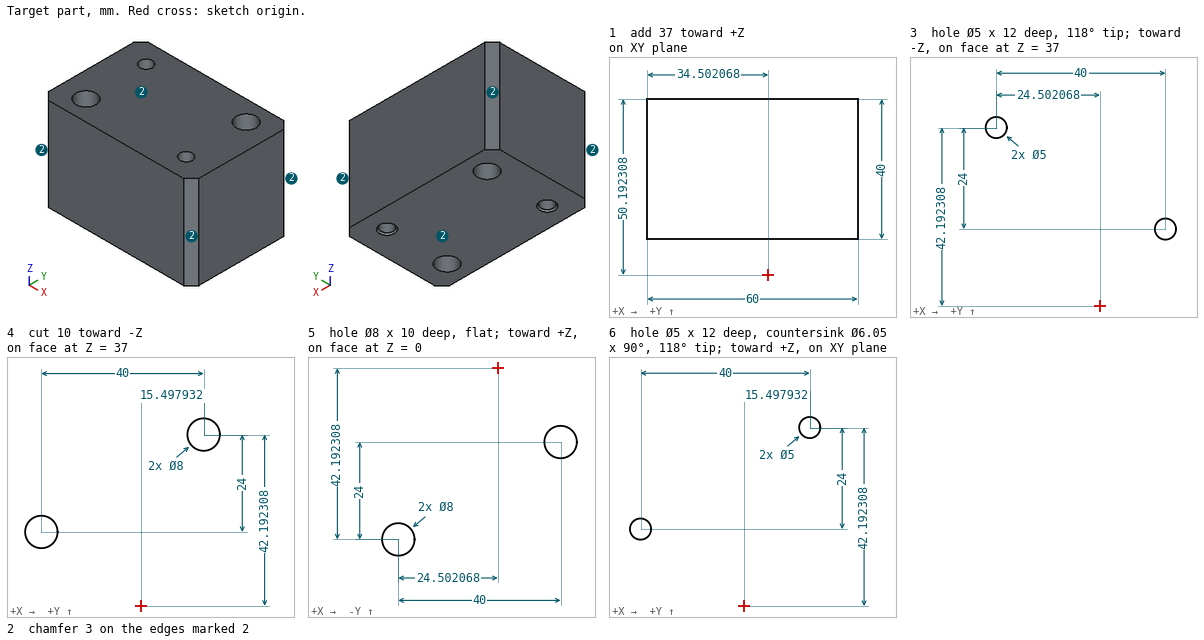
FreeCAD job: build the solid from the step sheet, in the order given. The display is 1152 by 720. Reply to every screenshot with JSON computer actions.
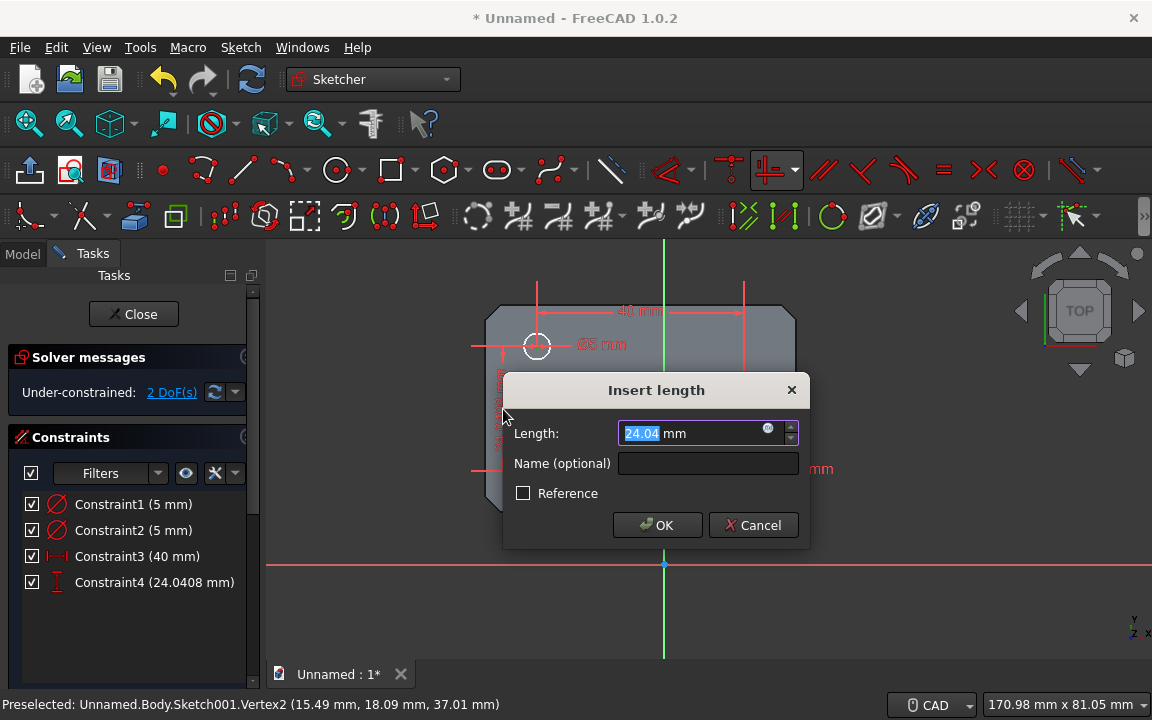
{"action": "type", "text": "24"}
{"action": "key", "text": "Return"}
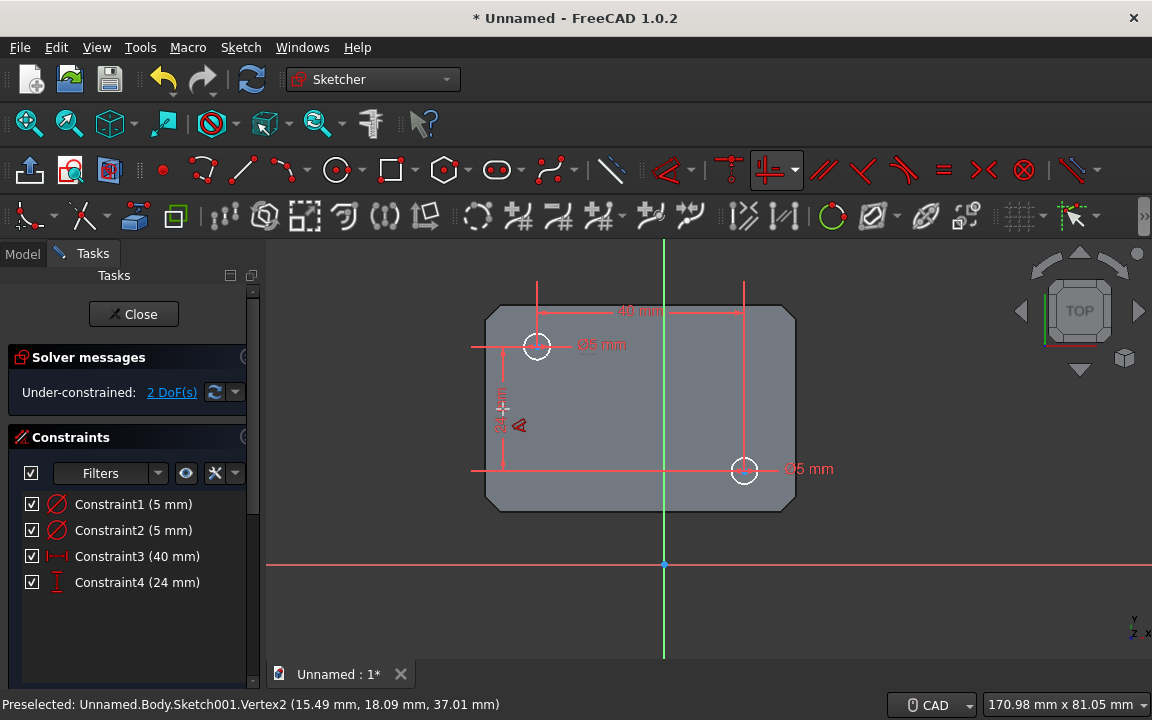
{"action": "left_click", "coordinate": [537, 347]}
{"action": "left_click", "coordinate": [601, 599]}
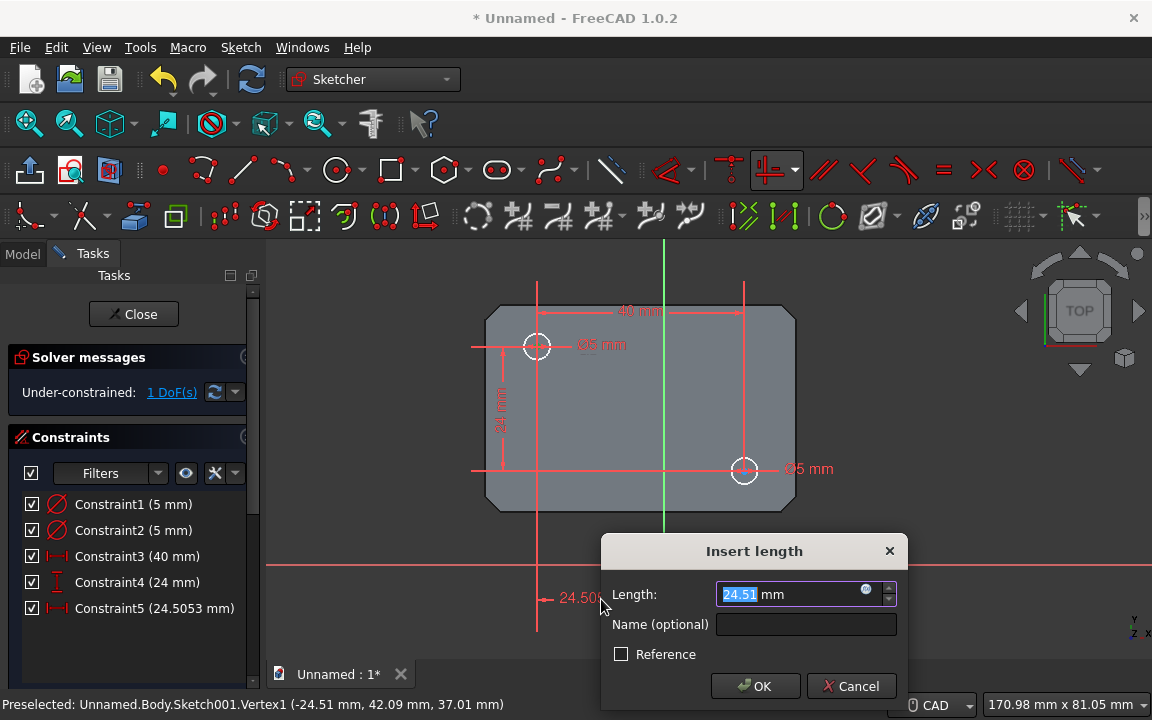
{"action": "type", "text": "24.502068"}
{"action": "key", "text": "Return"}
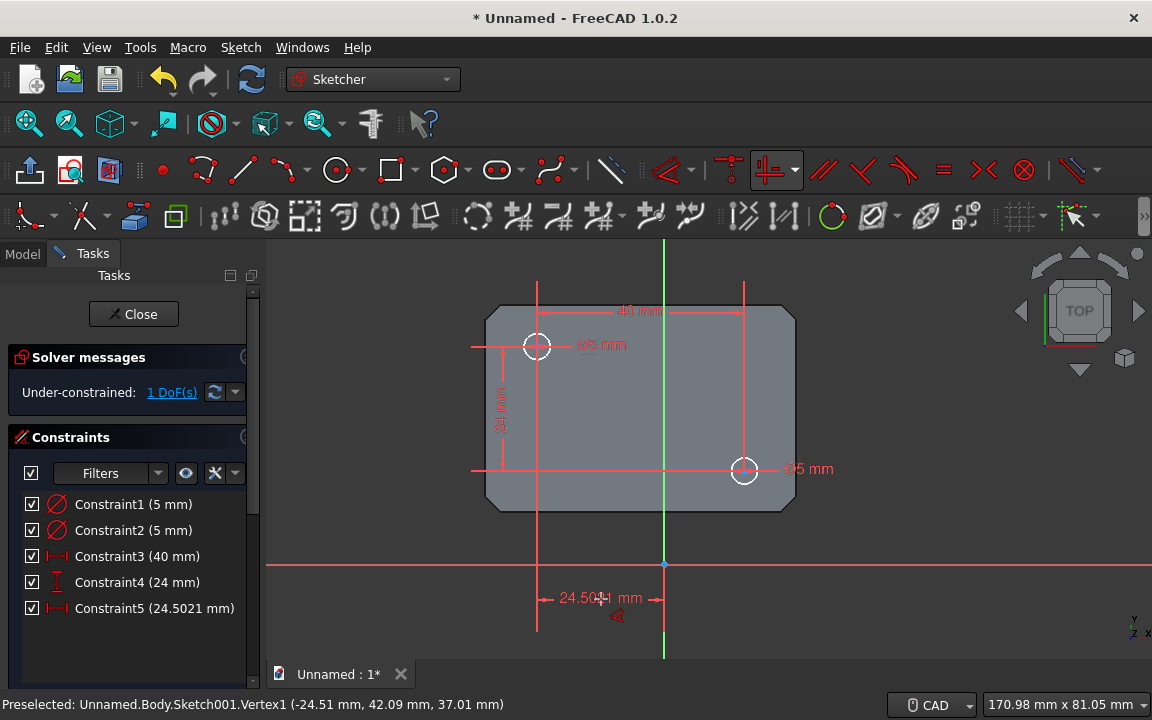
{"action": "left_click", "coordinate": [537, 347]}
{"action": "left_click", "coordinate": [503, 456]}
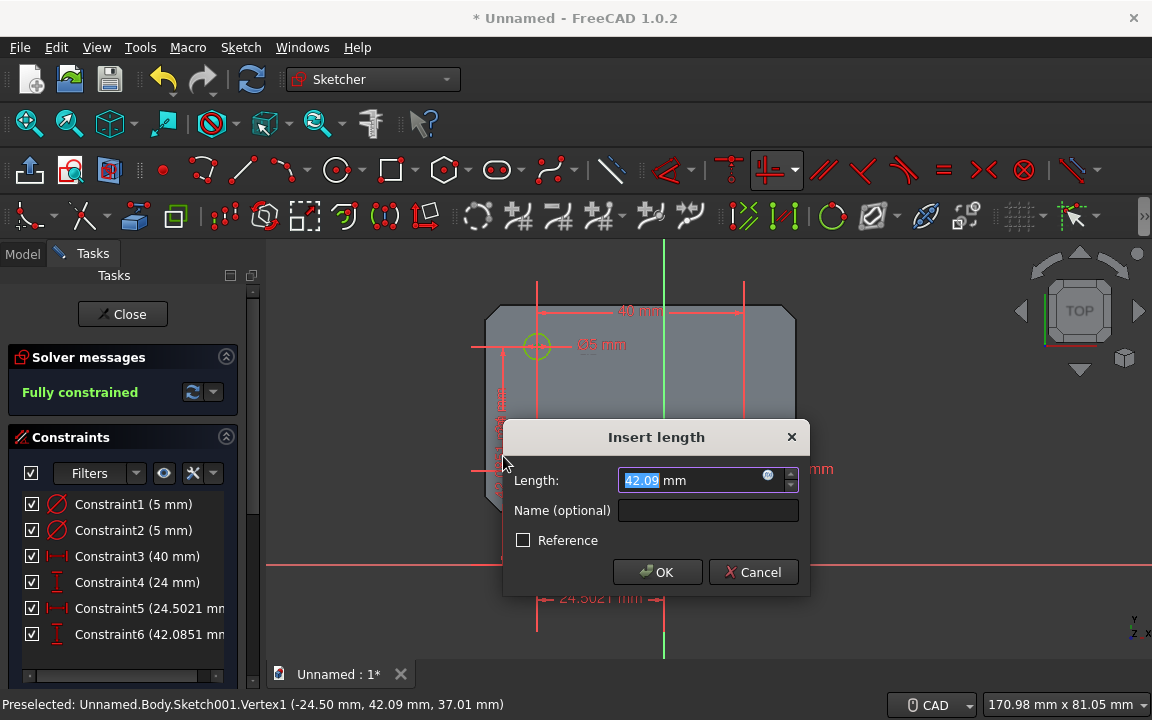
{"action": "type", "text": "42.192308"}
{"action": "key", "text": "Return"}
{"action": "key", "text": "Escape"}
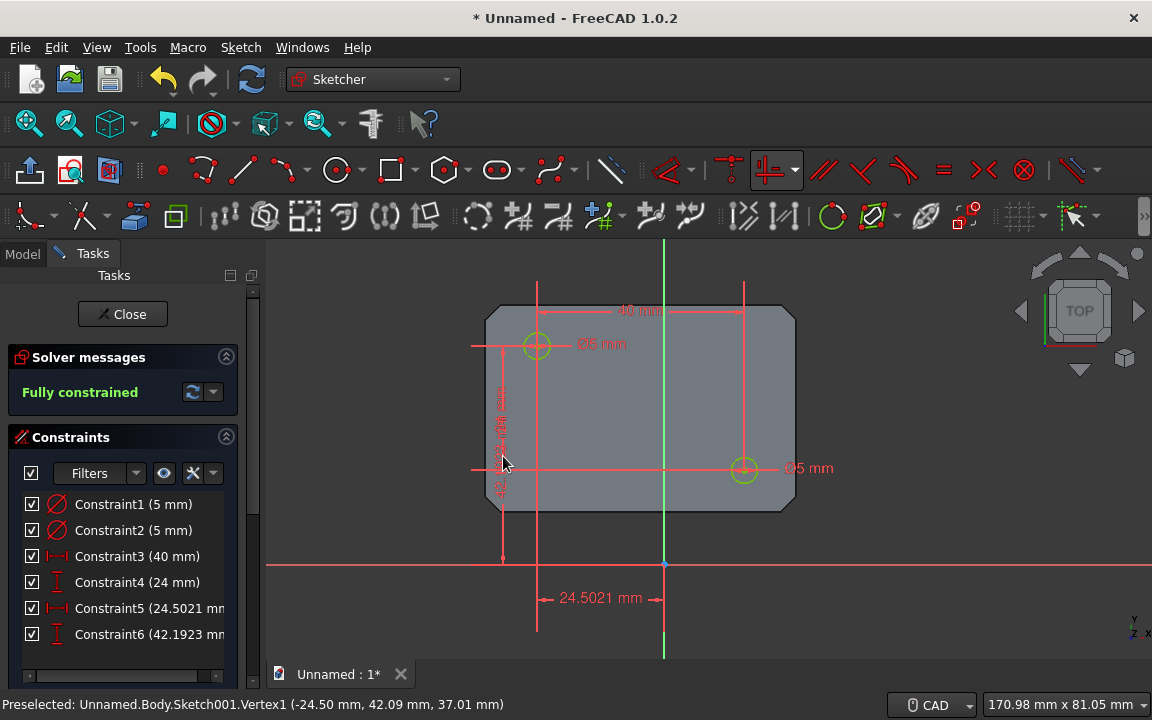
{"action": "left_click", "coordinate": [123, 314]}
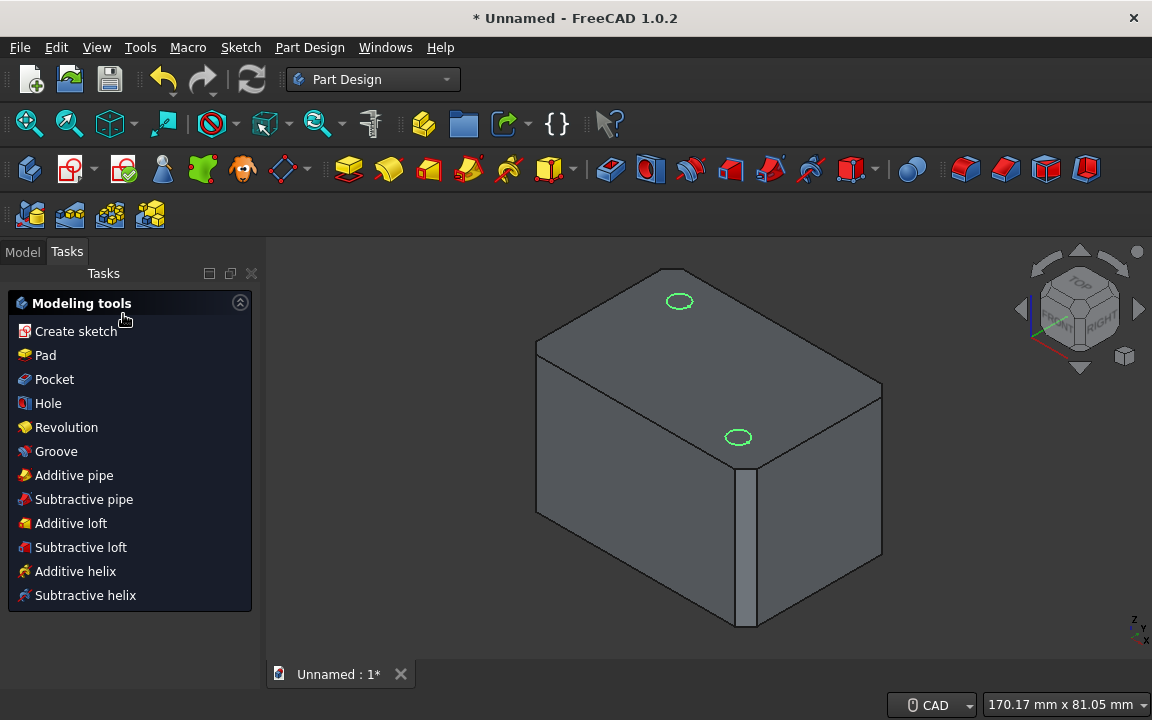
{"action": "left_click", "coordinate": [652, 170]}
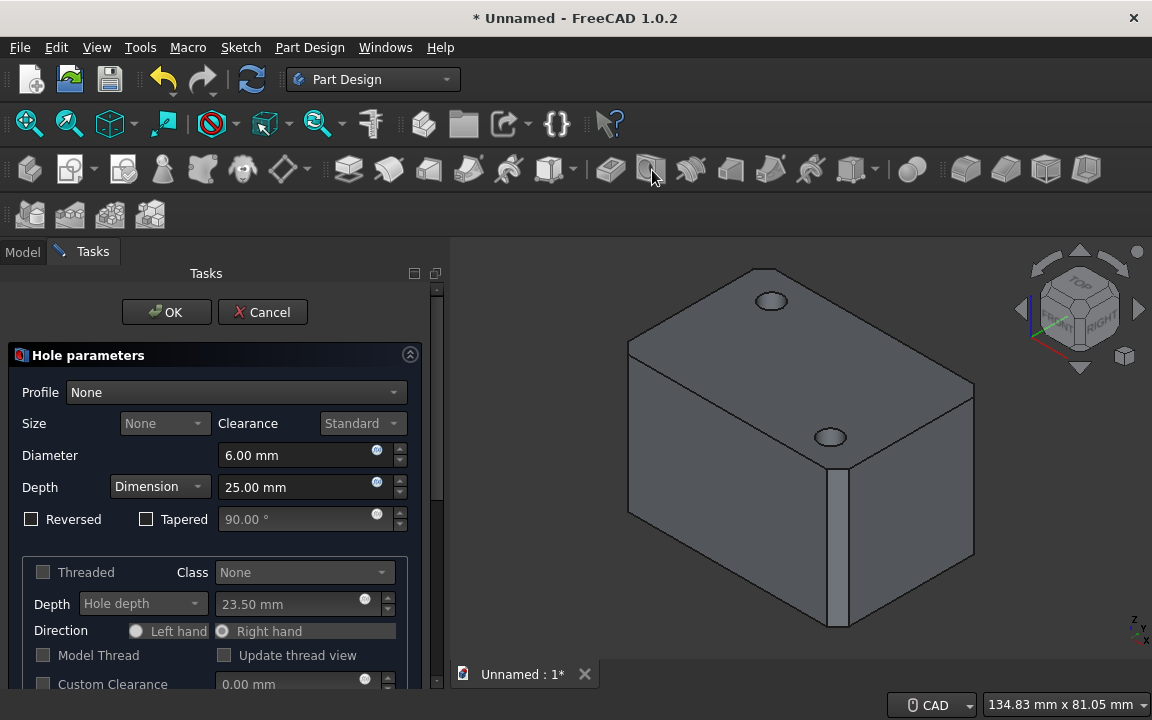
{"action": "triple_click", "coordinate": [305, 455]}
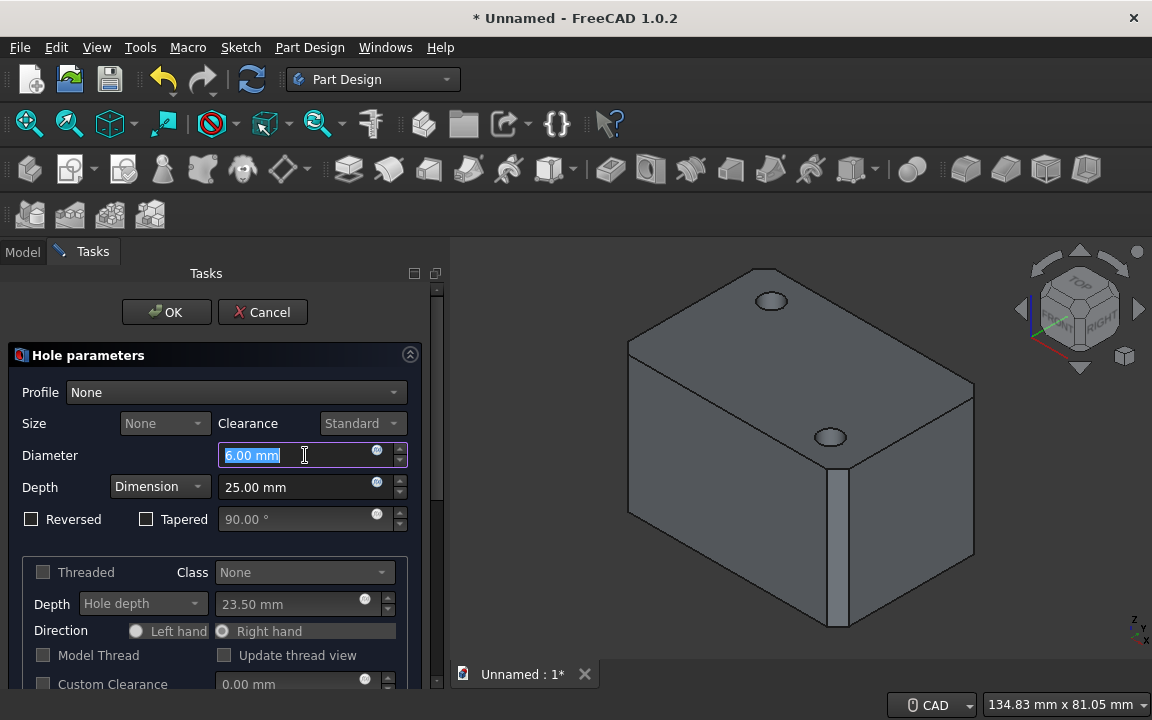
{"action": "type", "text": "5"}
{"action": "key", "text": "Tab"}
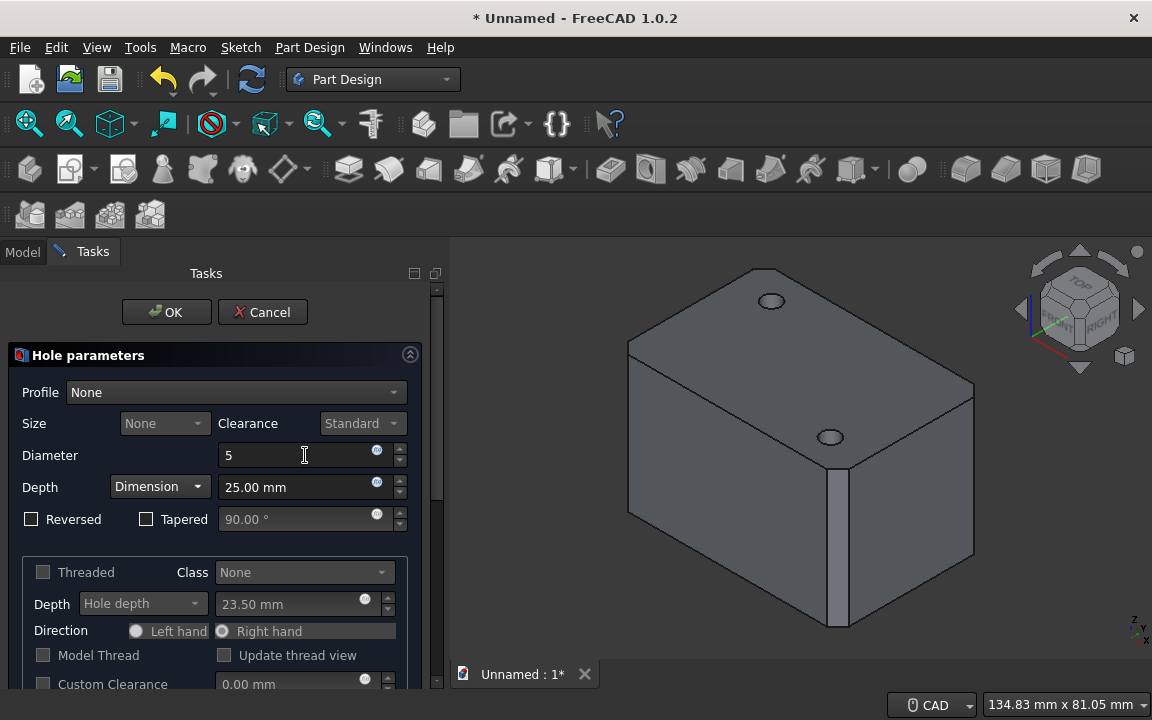
{"action": "triple_click", "coordinate": [305, 487]}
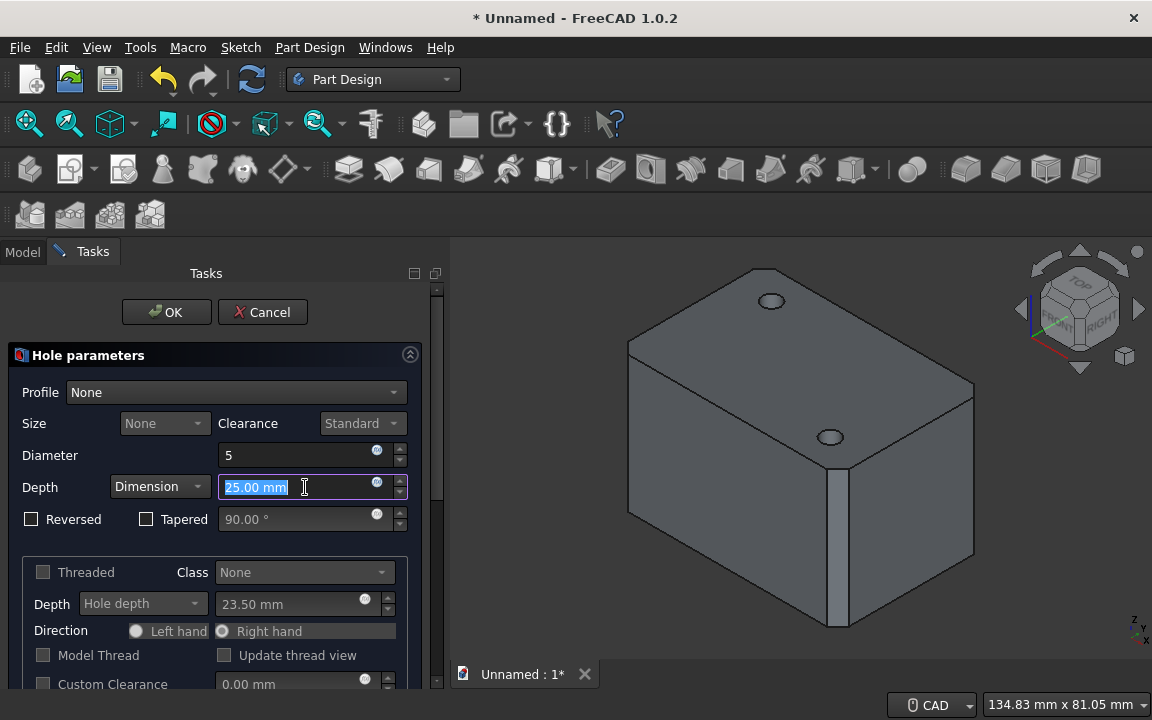
{"action": "type", "text": "12"}
{"action": "key", "text": "Tab"}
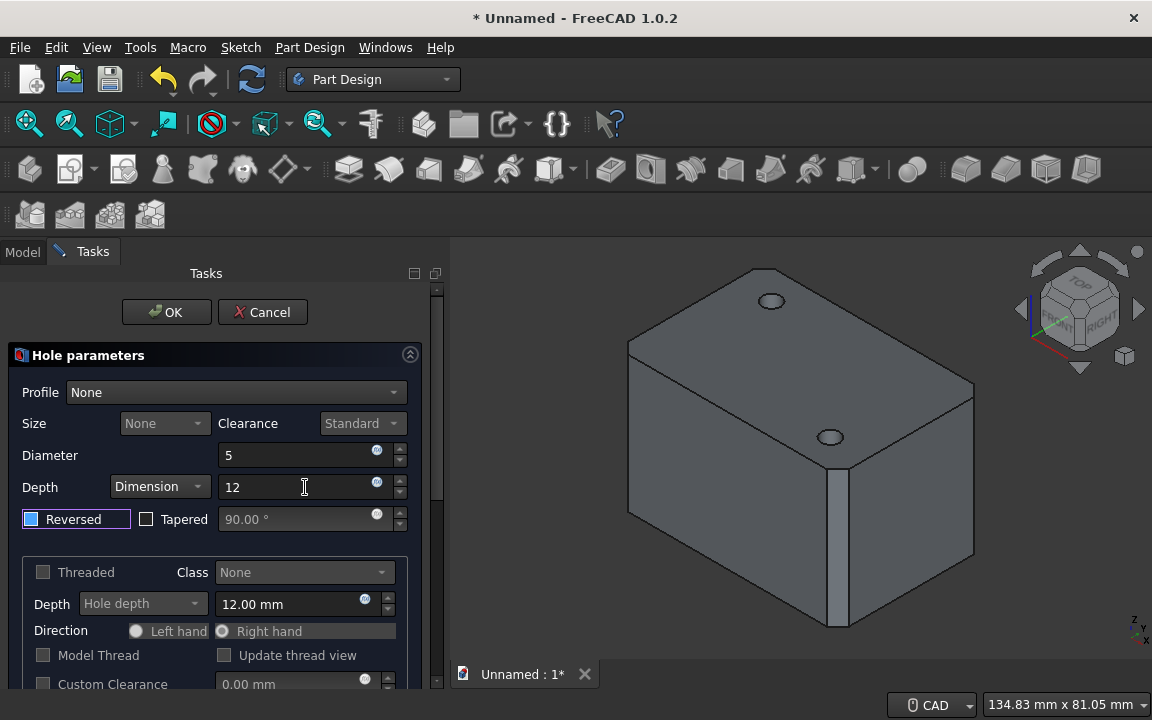
{"action": "left_click", "coordinate": [167, 312]}